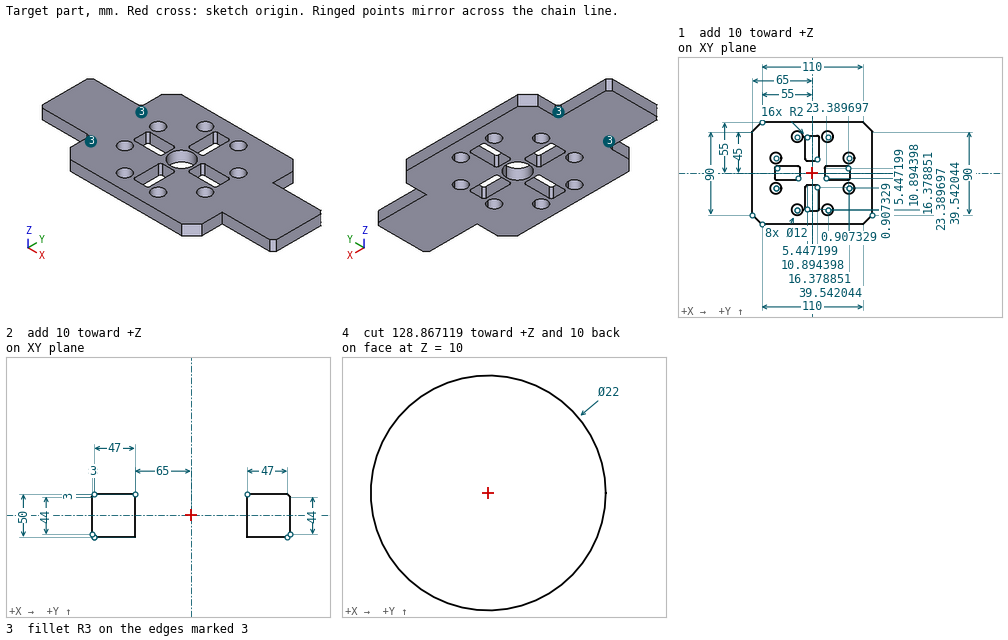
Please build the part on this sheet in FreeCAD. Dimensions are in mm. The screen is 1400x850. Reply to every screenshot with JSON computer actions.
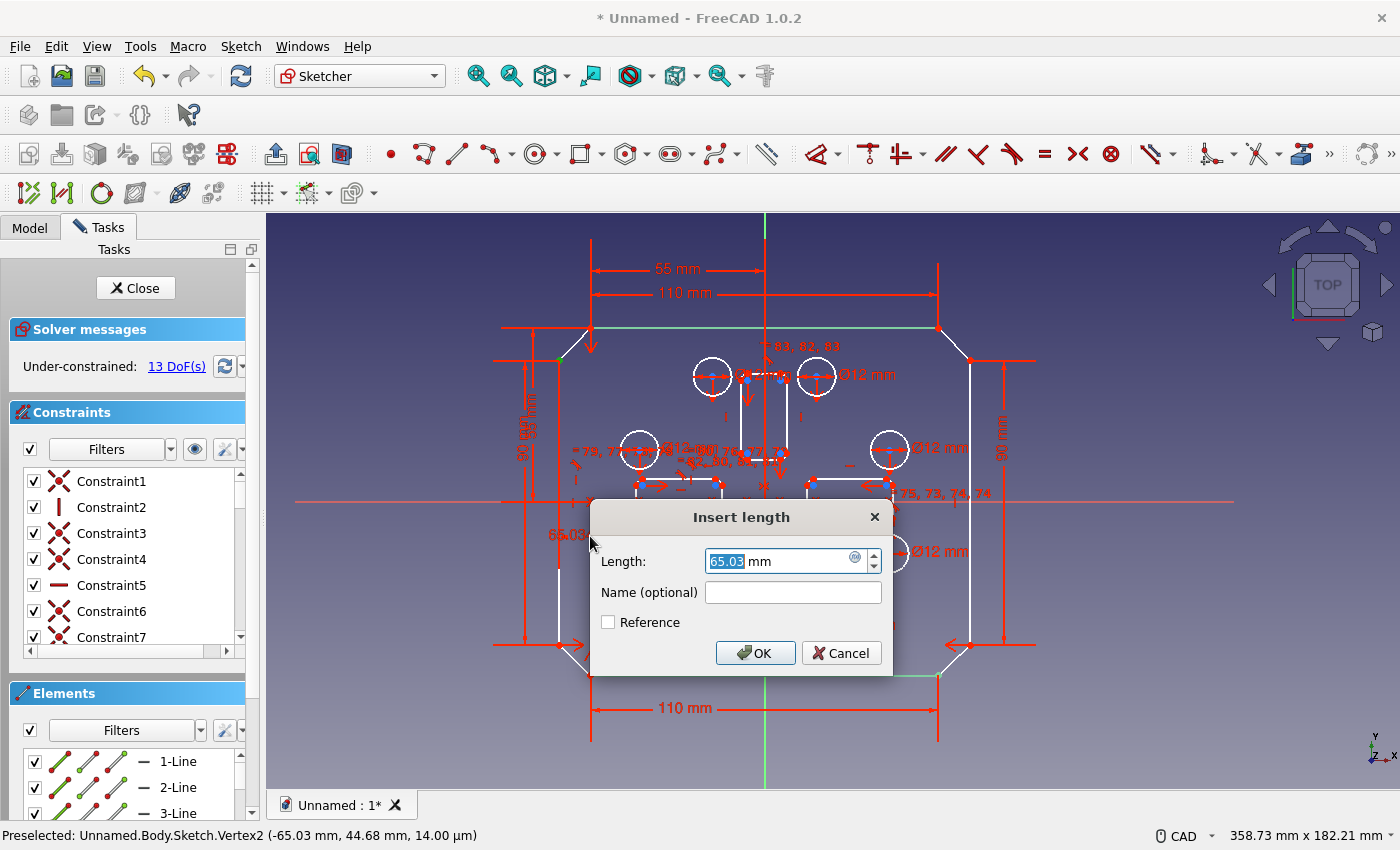
{"action": "type", "text": "65"}
{"action": "key", "text": "Return"}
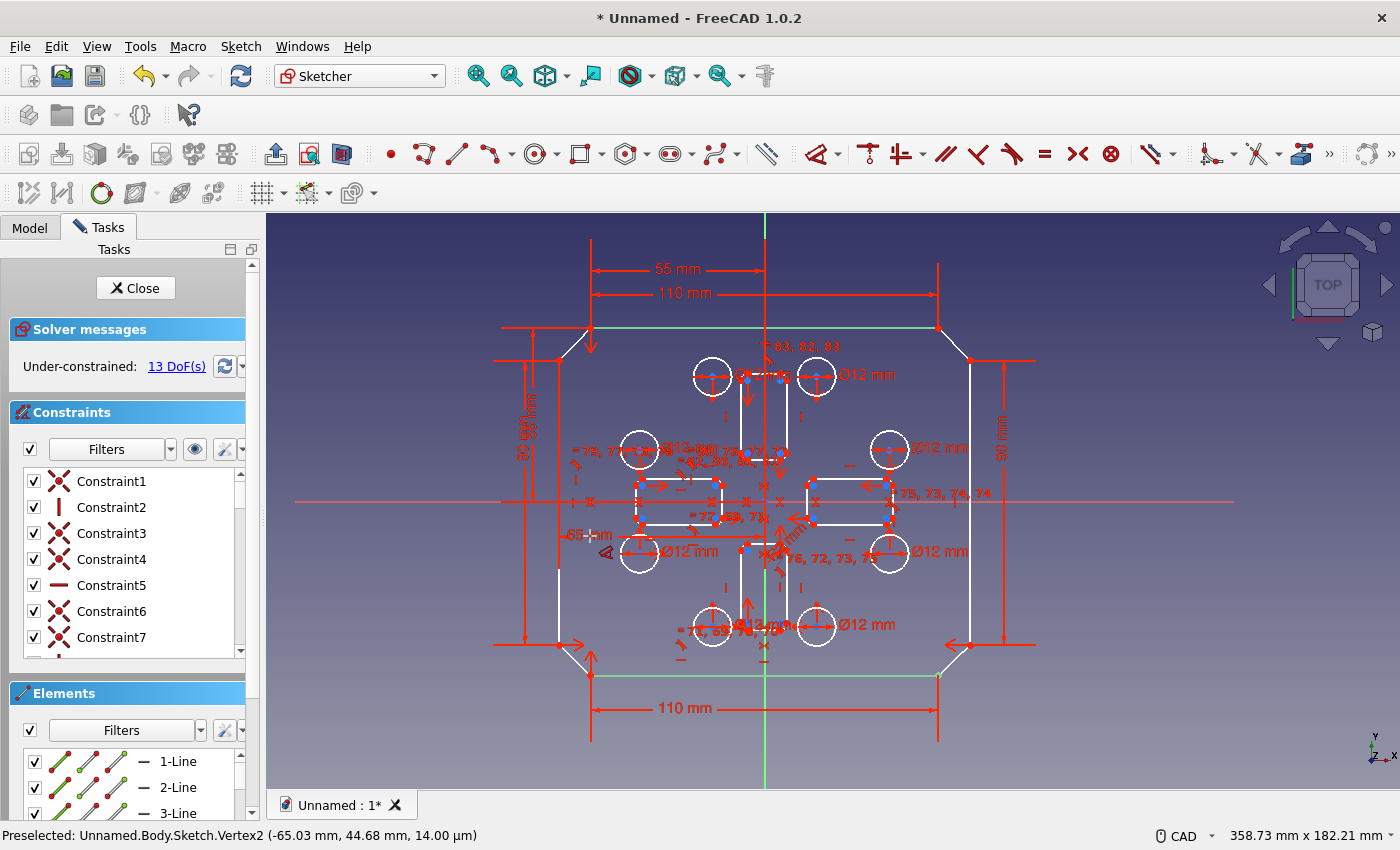
{"action": "left_click", "coordinate": [559, 361]}
{"action": "left_click", "coordinate": [525, 464]}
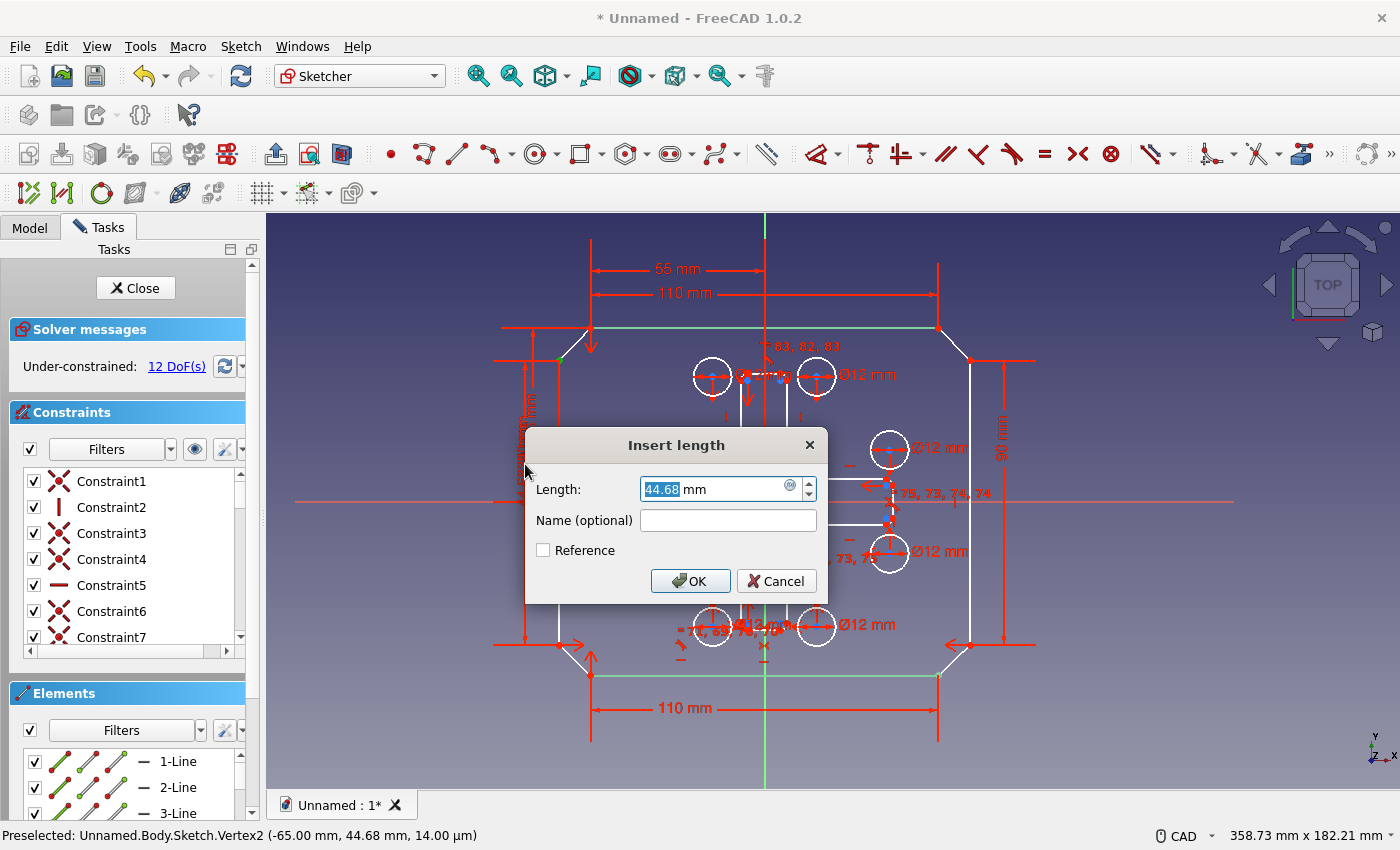
{"action": "type", "text": "45"}
{"action": "key", "text": "Return"}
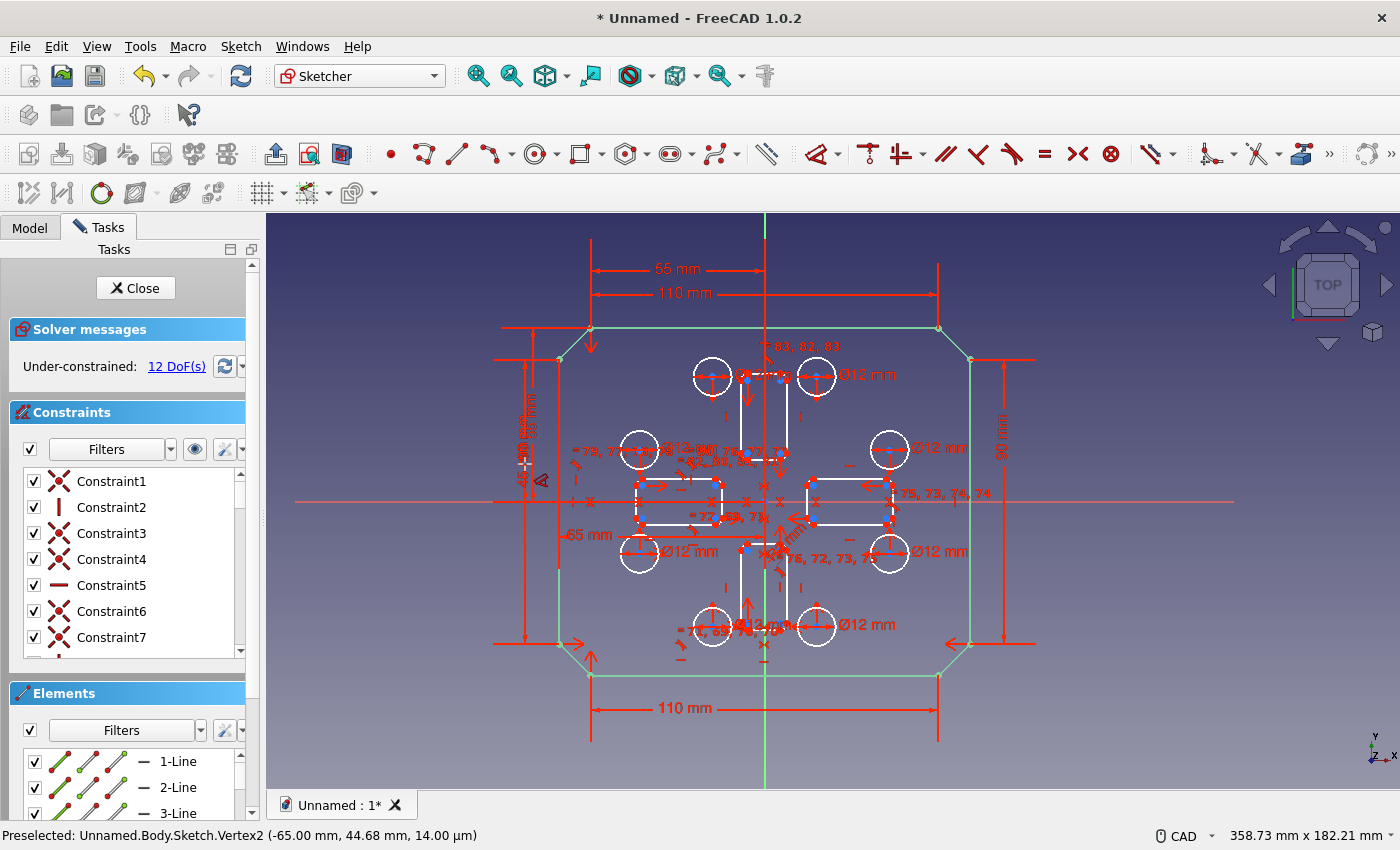
{"action": "left_click", "coordinate": [761, 544]}
{"action": "left_click", "coordinate": [756, 578]}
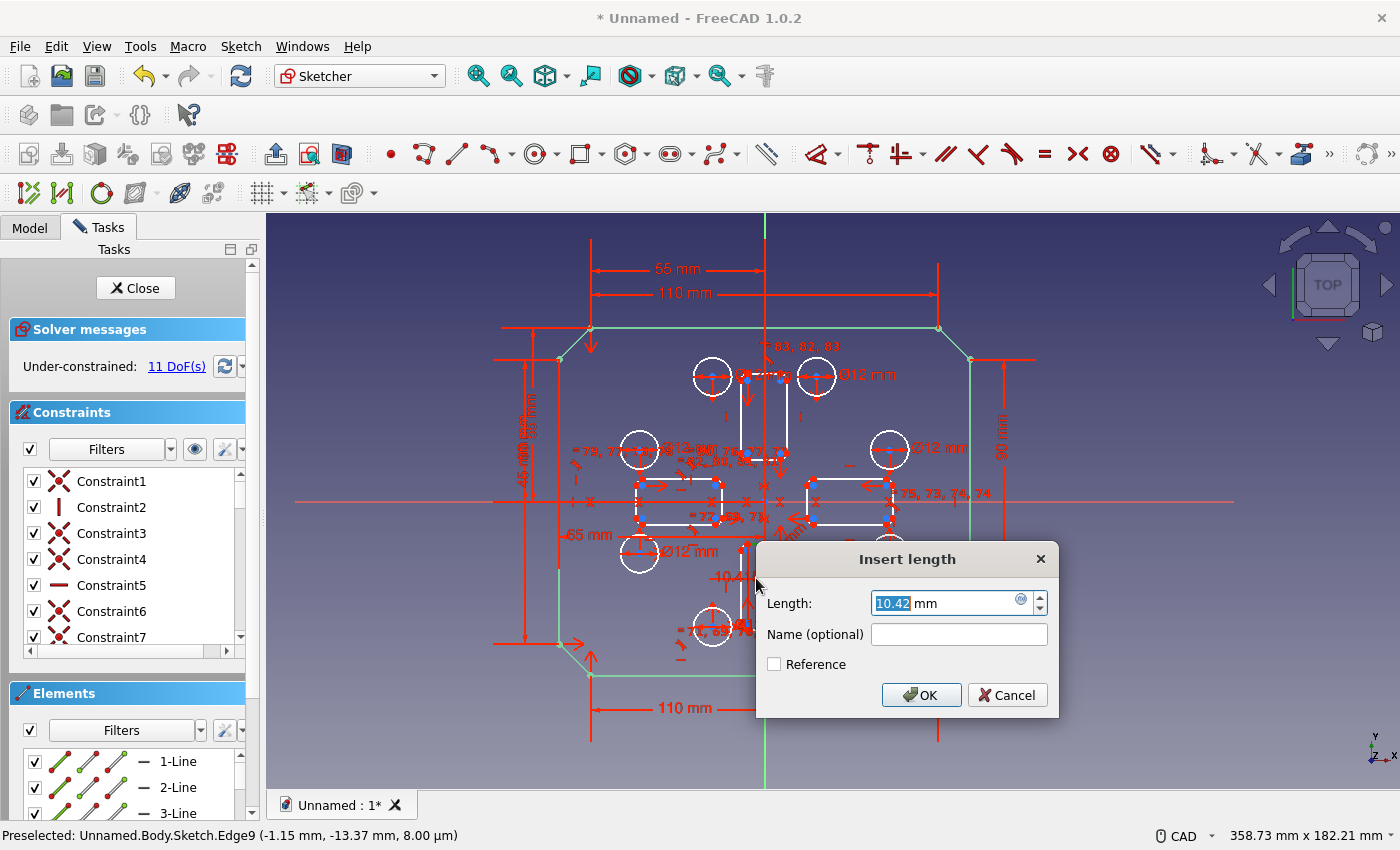
{"action": "type", "text": "10.894398"}
{"action": "key", "text": "Return"}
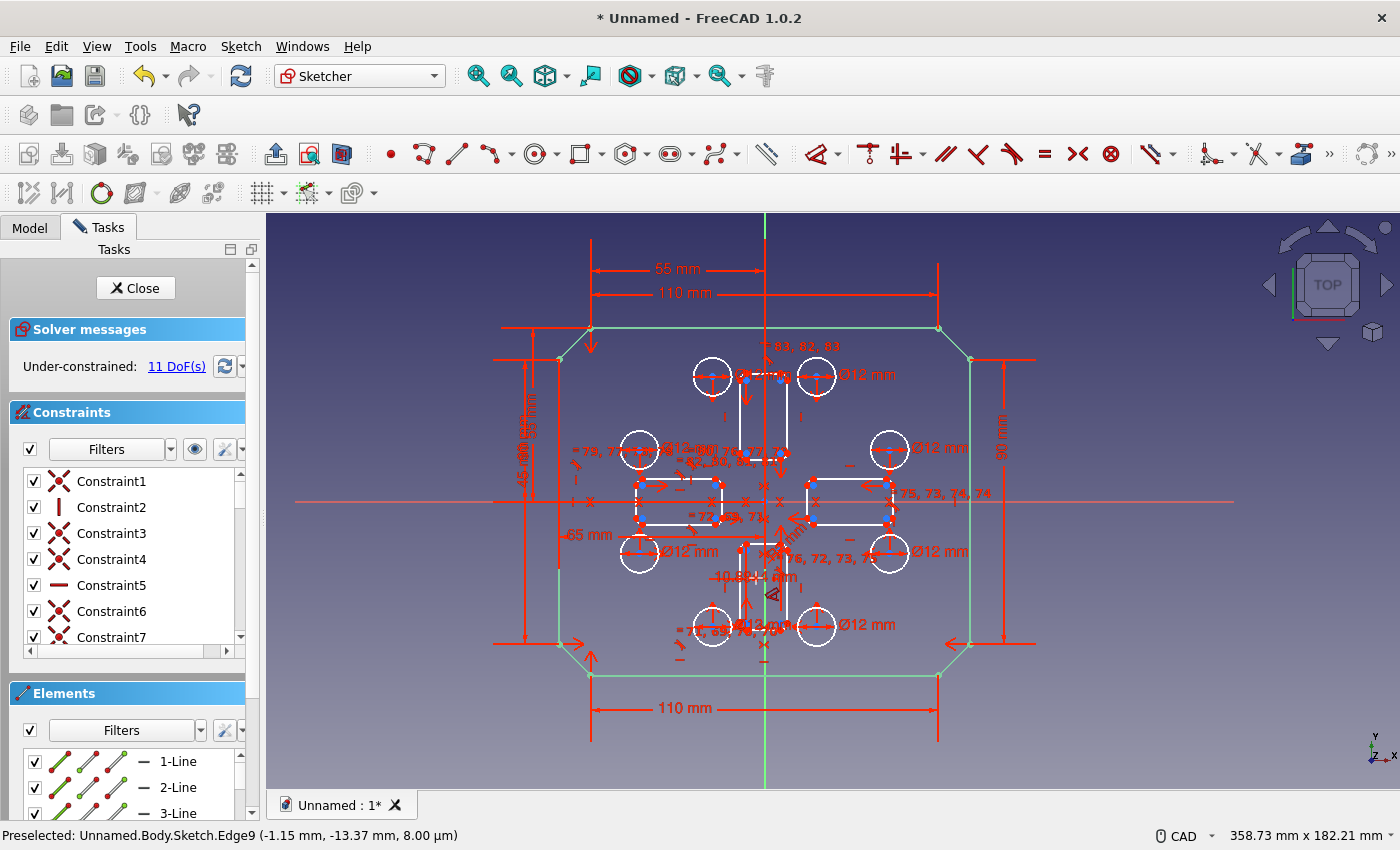
{"action": "left_click", "coordinate": [787, 572]}
{"action": "left_click", "coordinate": [845, 587]}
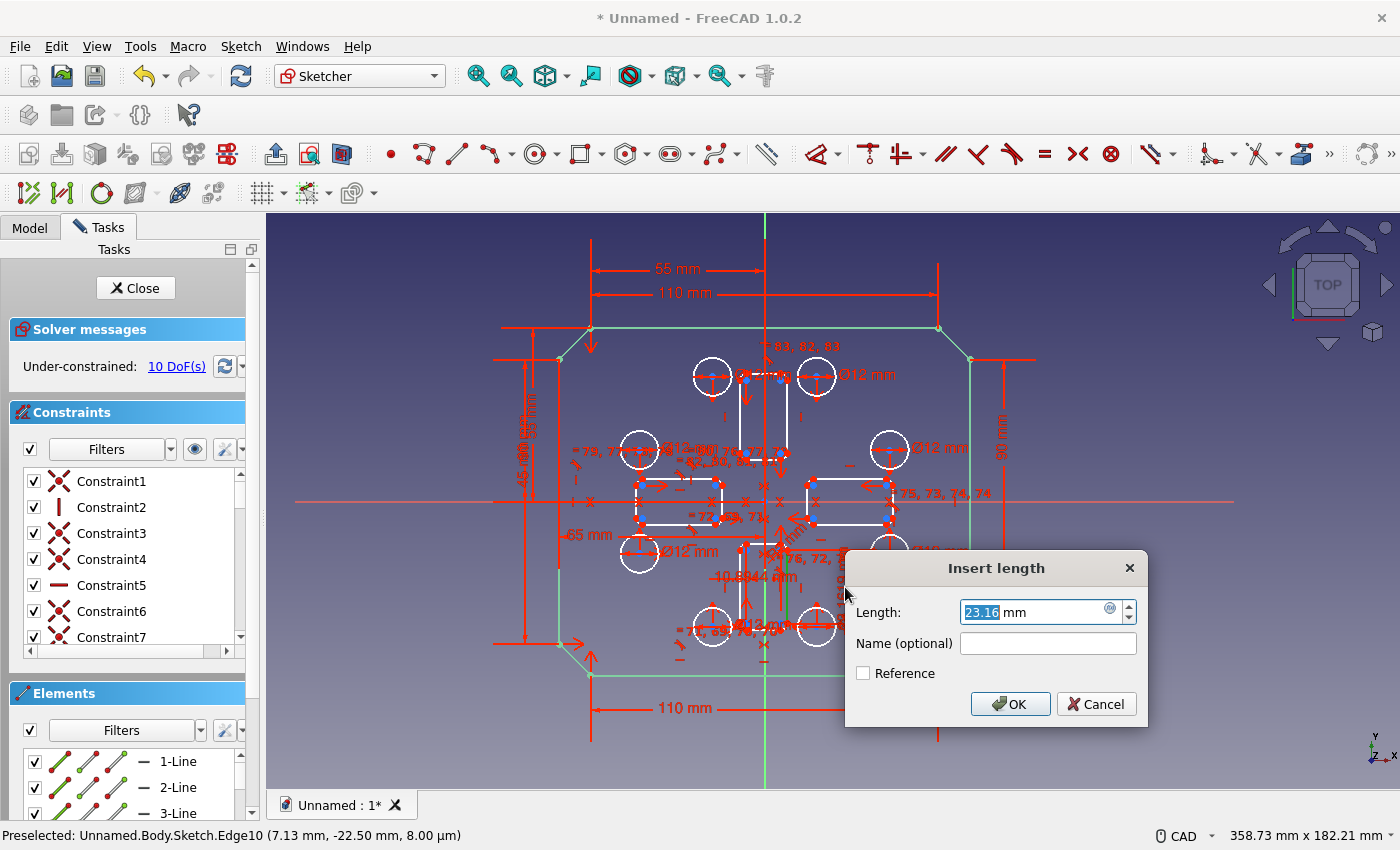
{"action": "type", "text": "23.389697"}
{"action": "key", "text": "Return"}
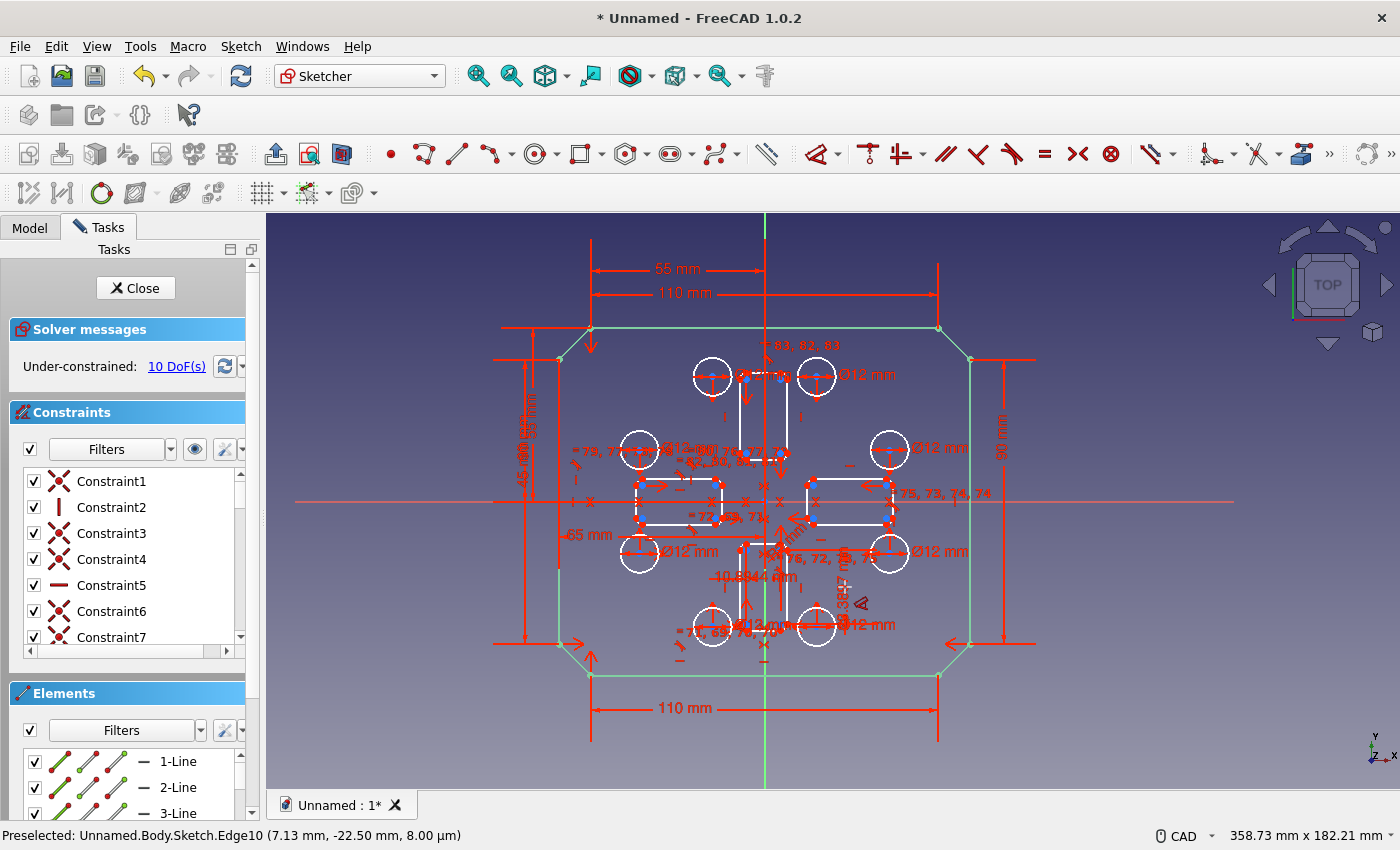
{"action": "left_click", "coordinate": [807, 505]}
{"action": "left_click", "coordinate": [841, 495]}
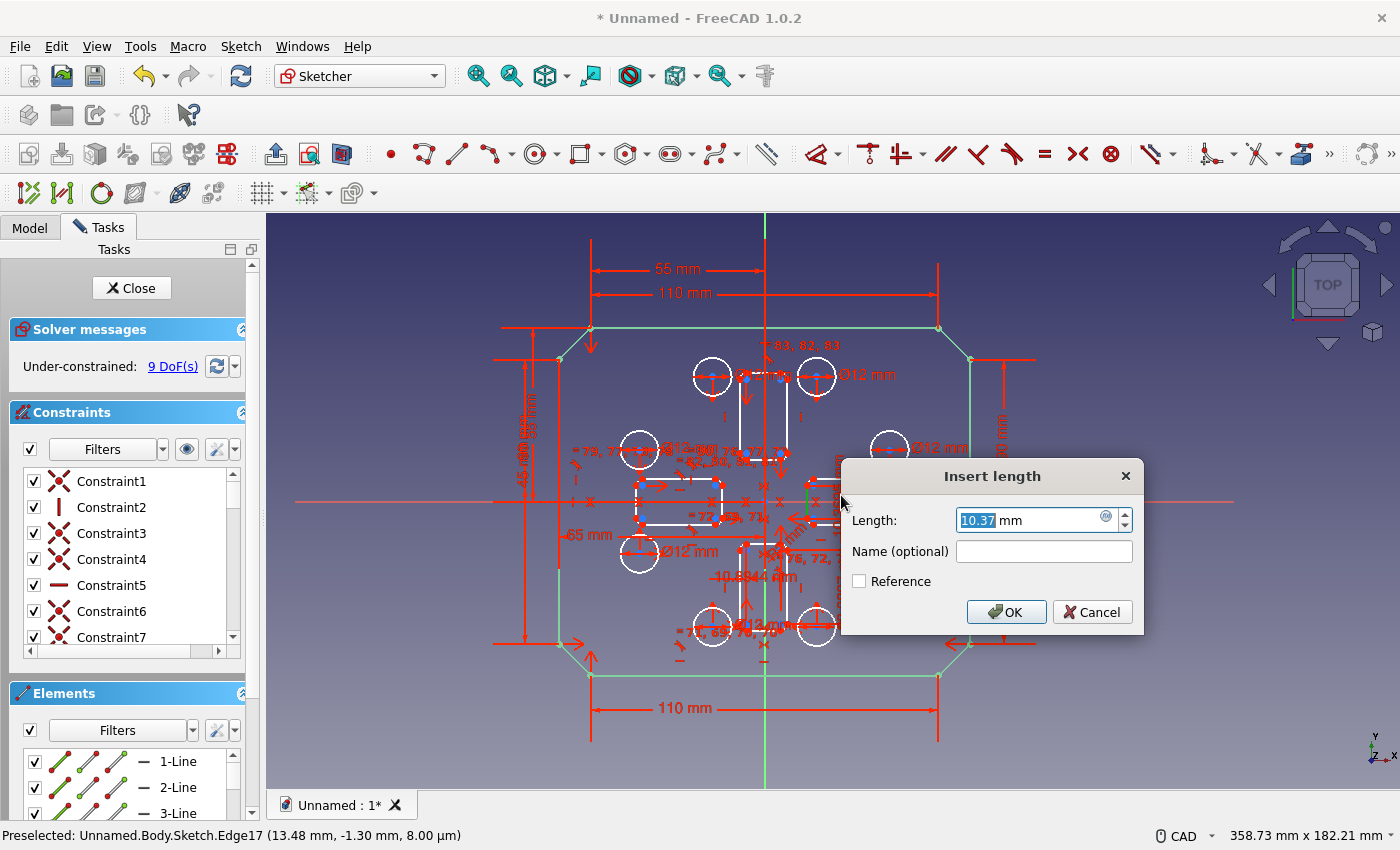
{"action": "type", "text": "10.894398"}
{"action": "key", "text": "Return"}